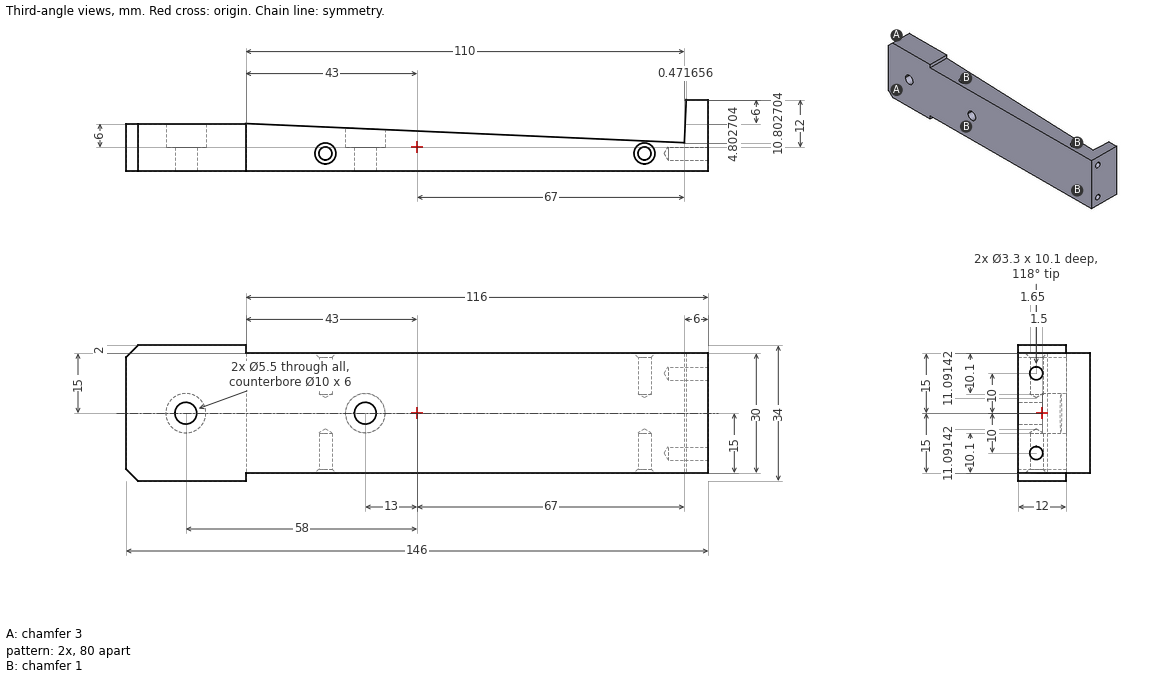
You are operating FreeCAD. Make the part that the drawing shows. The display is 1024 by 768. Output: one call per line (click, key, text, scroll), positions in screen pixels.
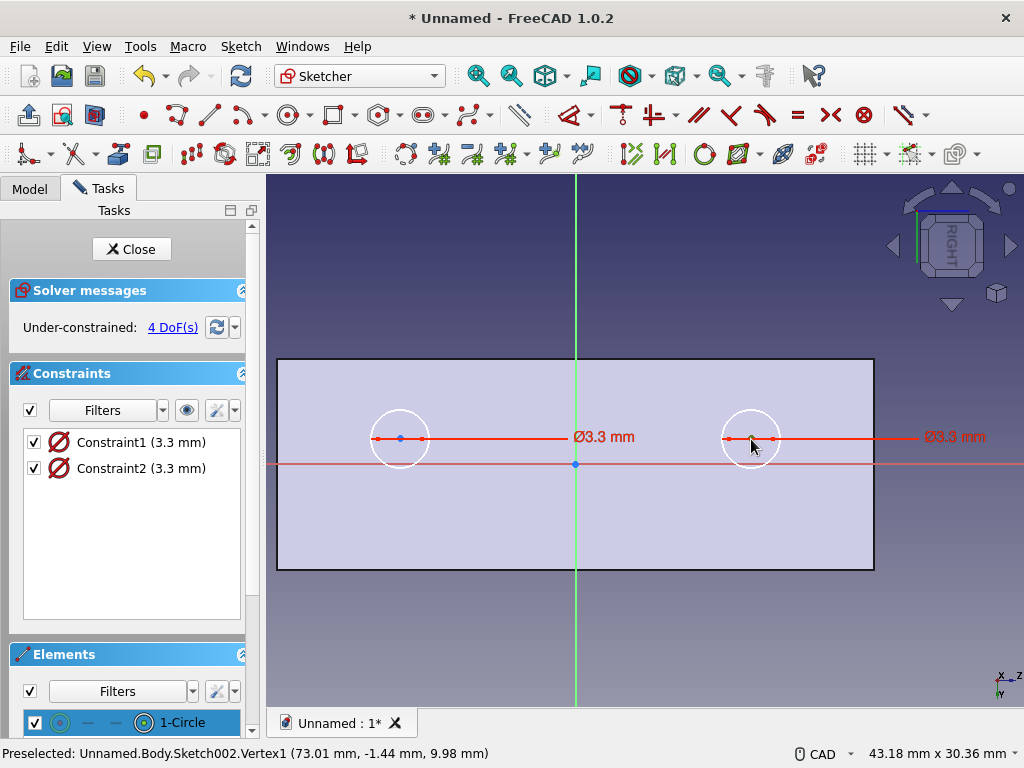
click(400, 439)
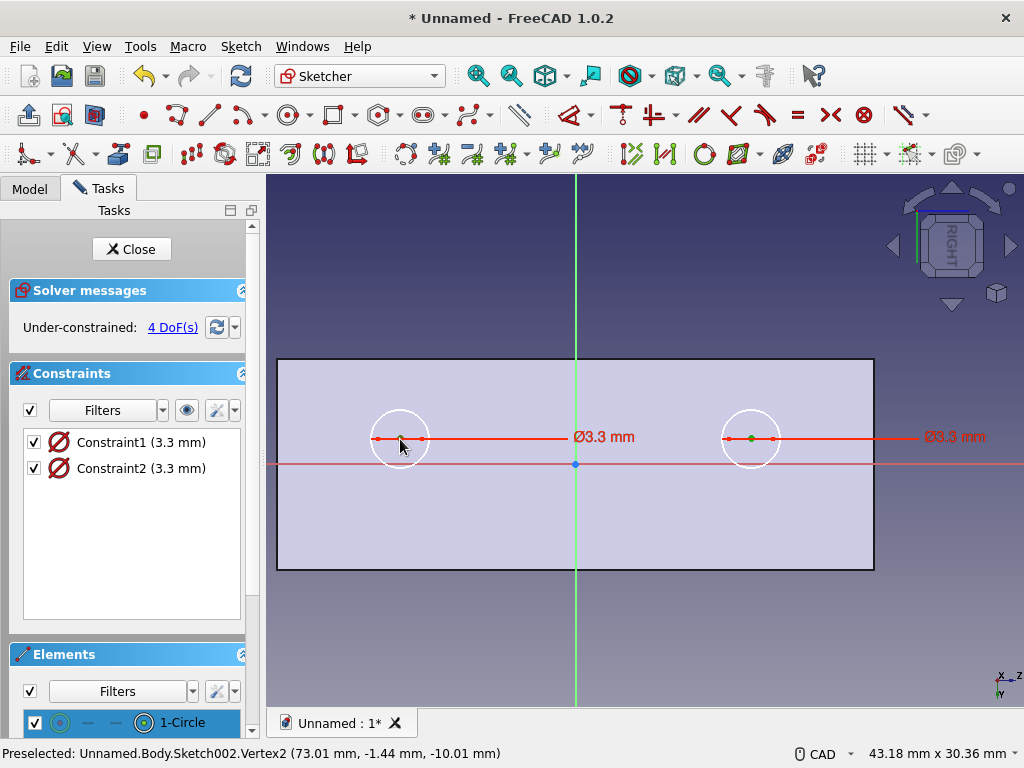
click(676, 116)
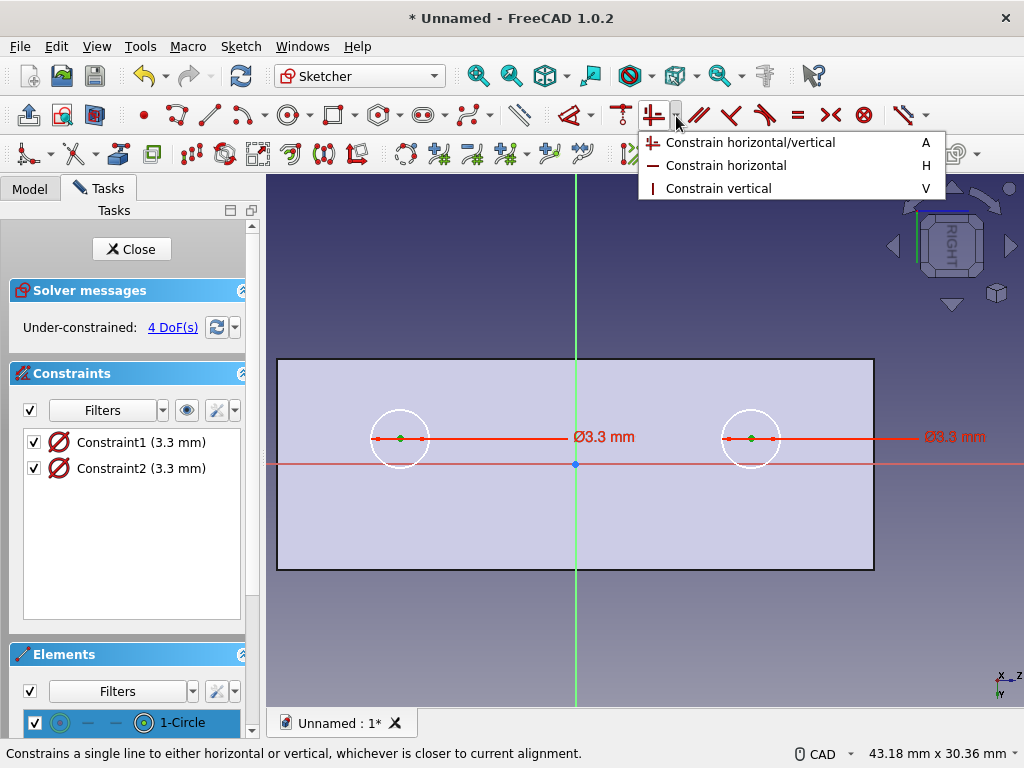
click(792, 166)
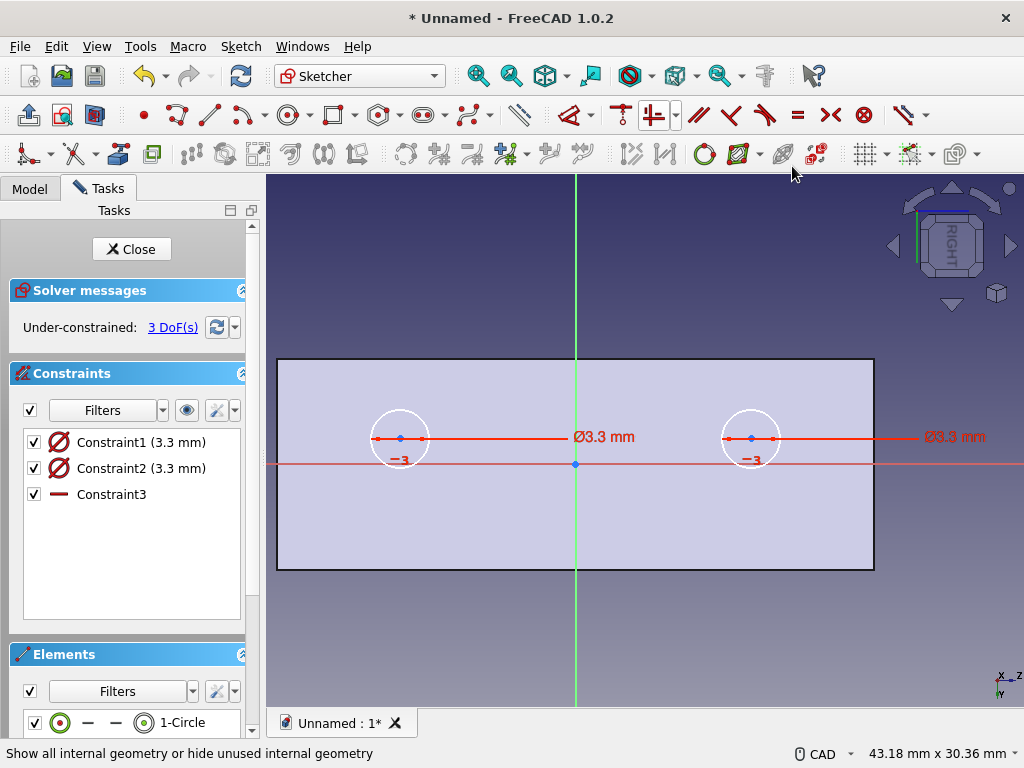
key(d)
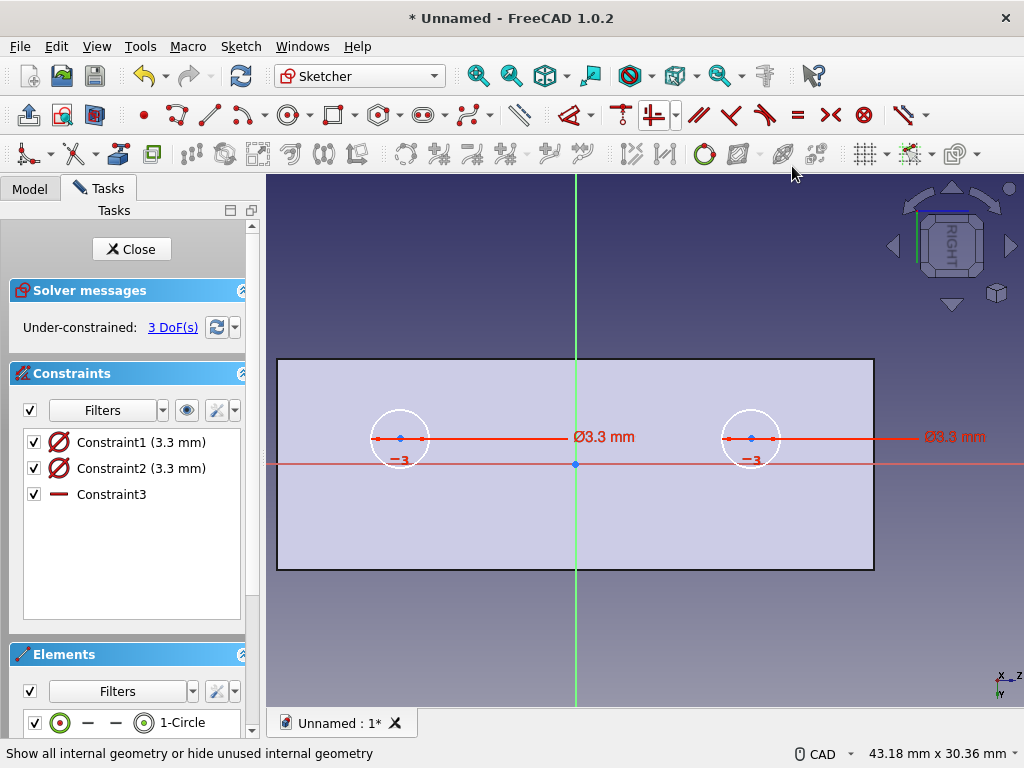
click(751, 439)
click(663, 498)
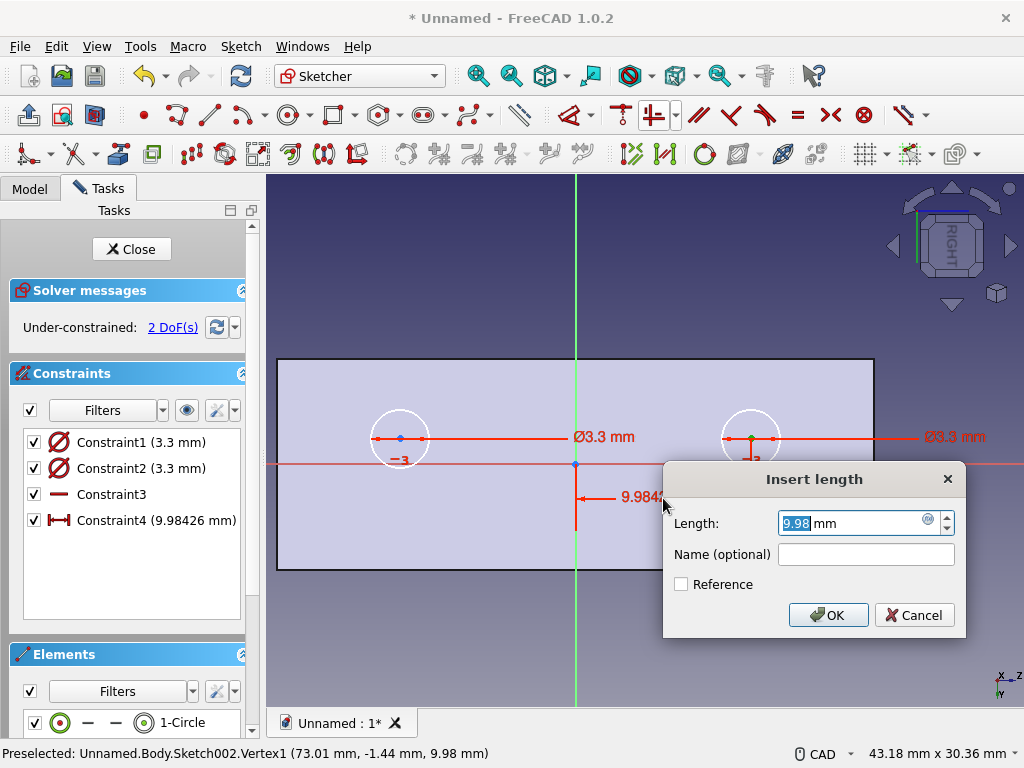
text(10)
key(Return)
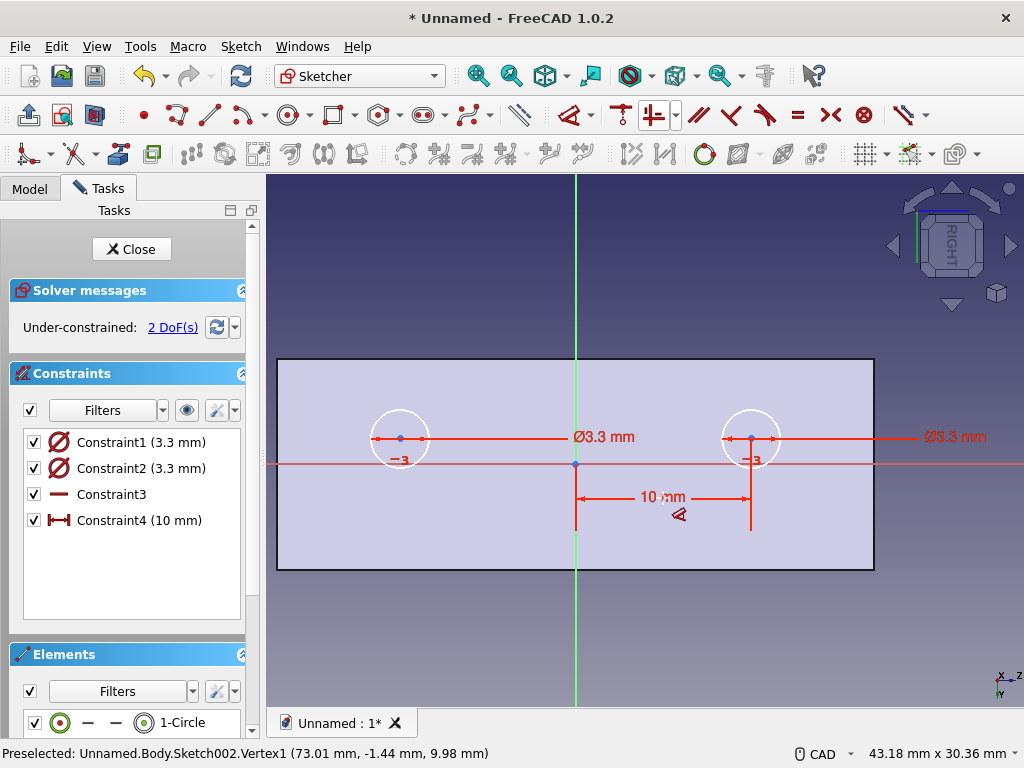
click(400, 439)
click(488, 498)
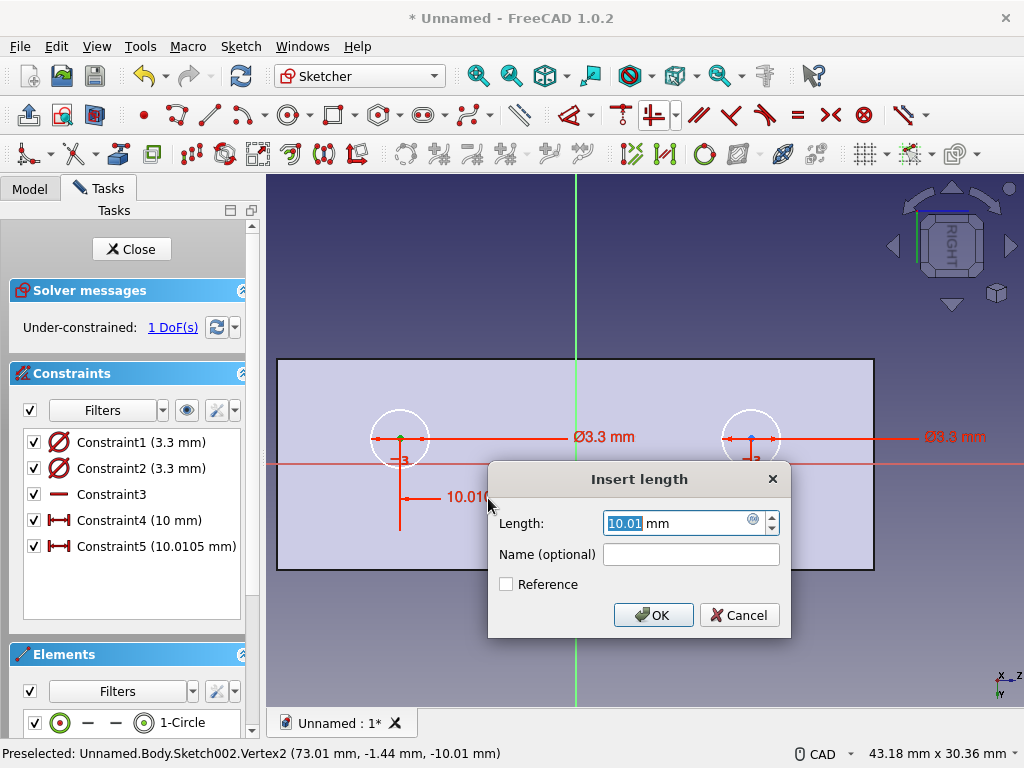
text(10)
key(Return)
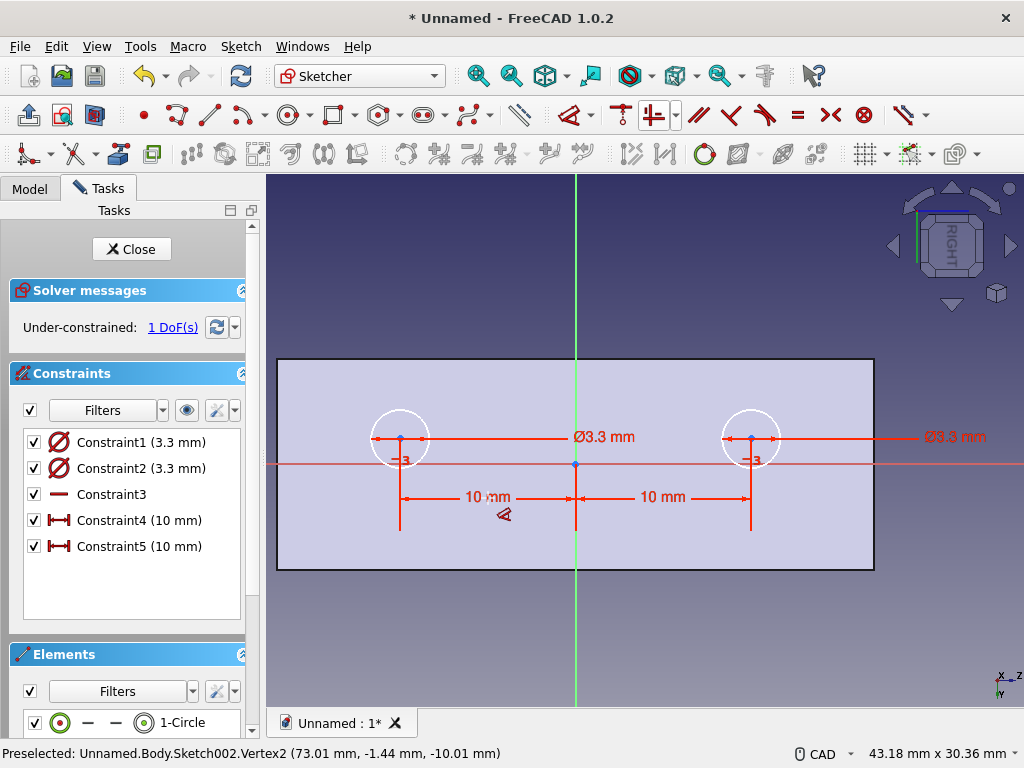
scroll(751, 439, up, 3)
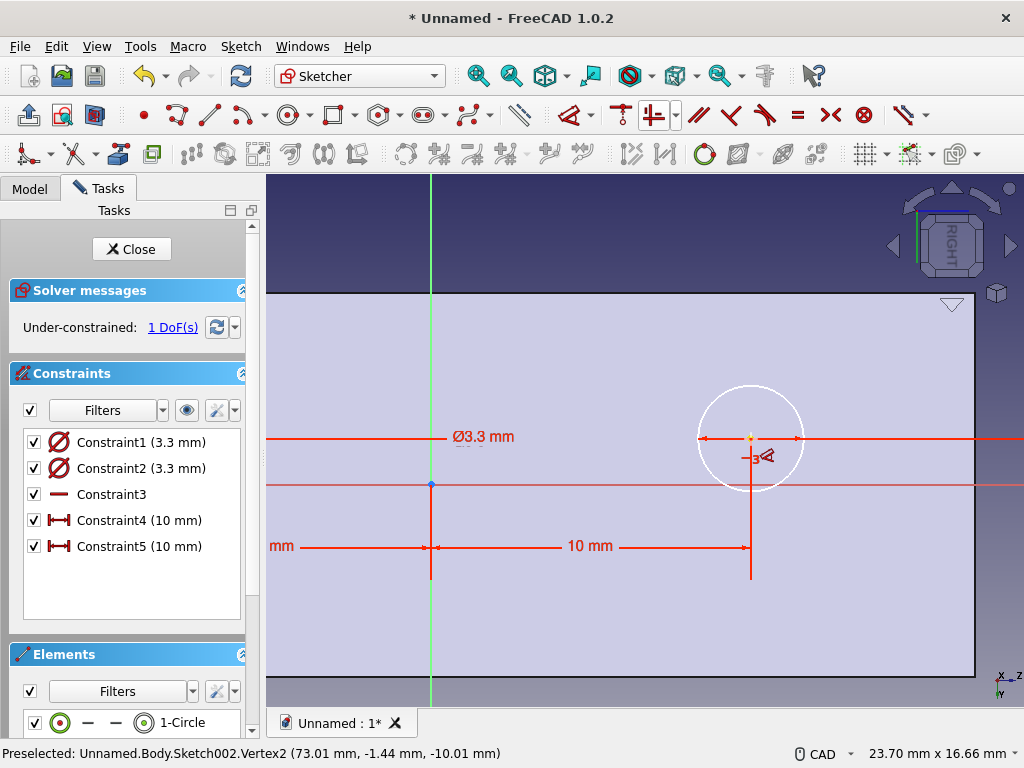
click(751, 439)
click(785, 451)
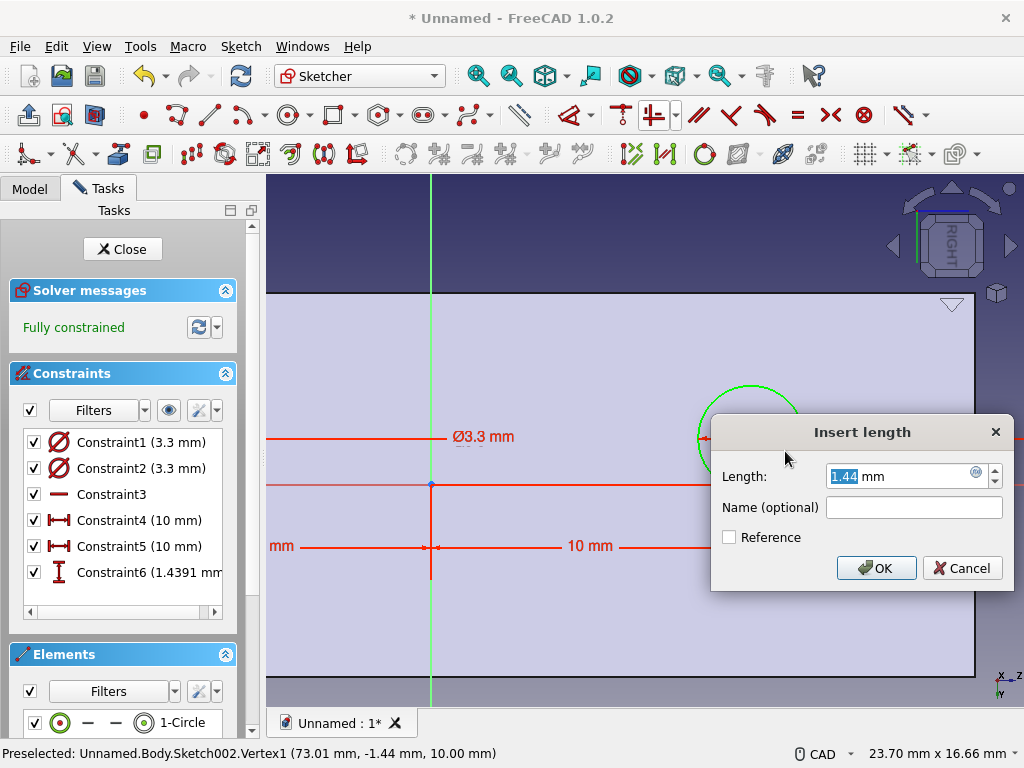
text(1.5)
key(Return)
key(Escape)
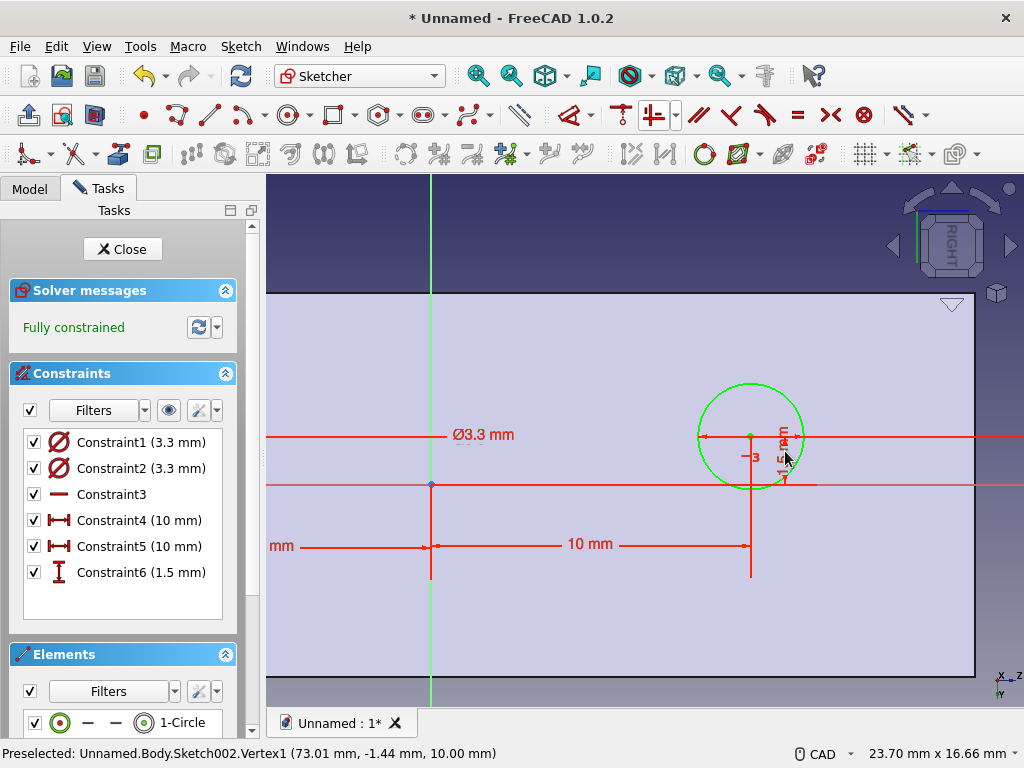
click(123, 249)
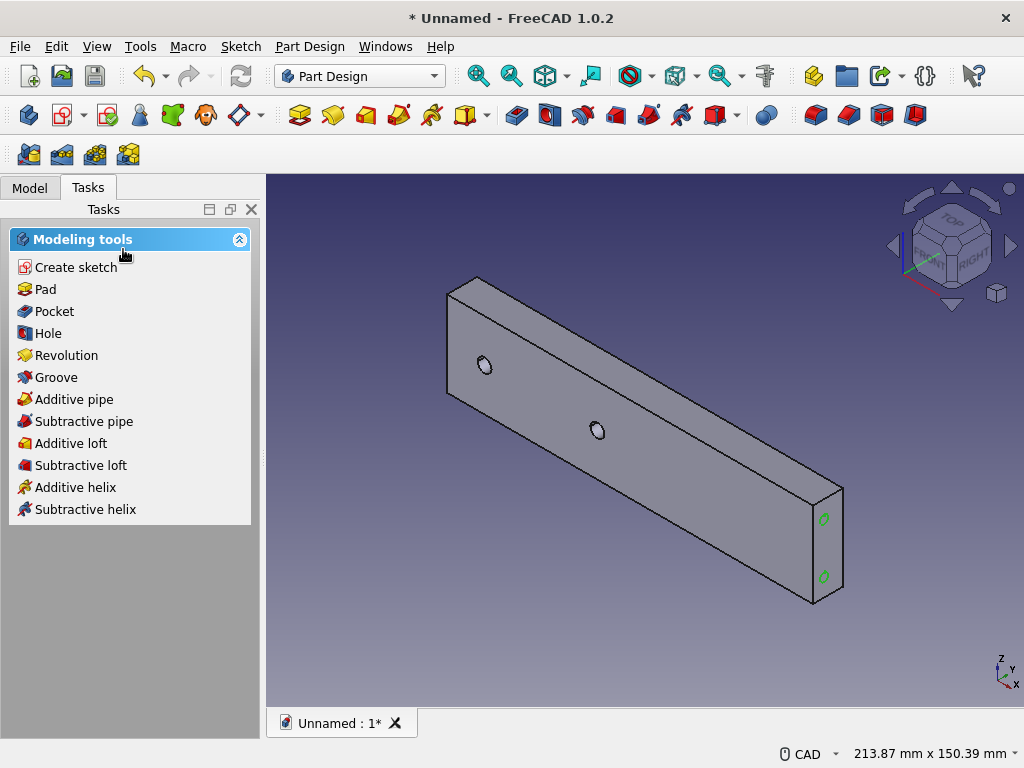
click(550, 116)